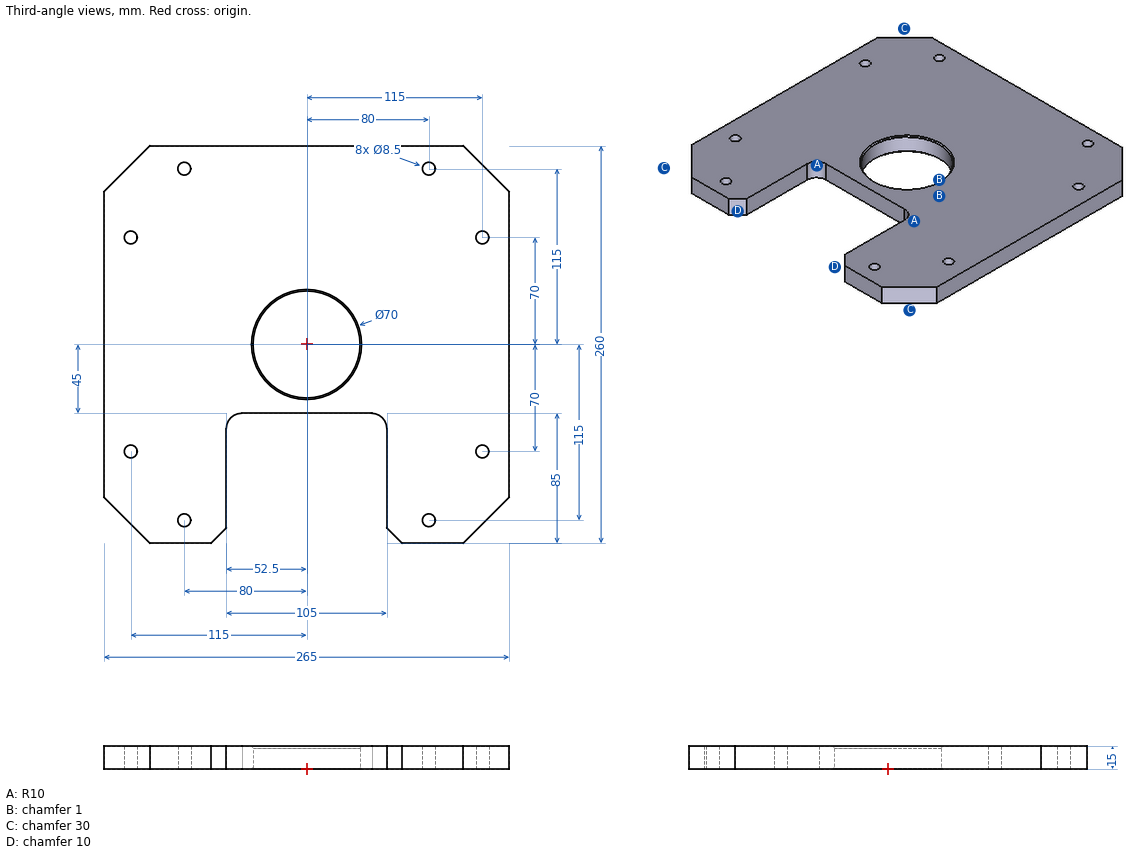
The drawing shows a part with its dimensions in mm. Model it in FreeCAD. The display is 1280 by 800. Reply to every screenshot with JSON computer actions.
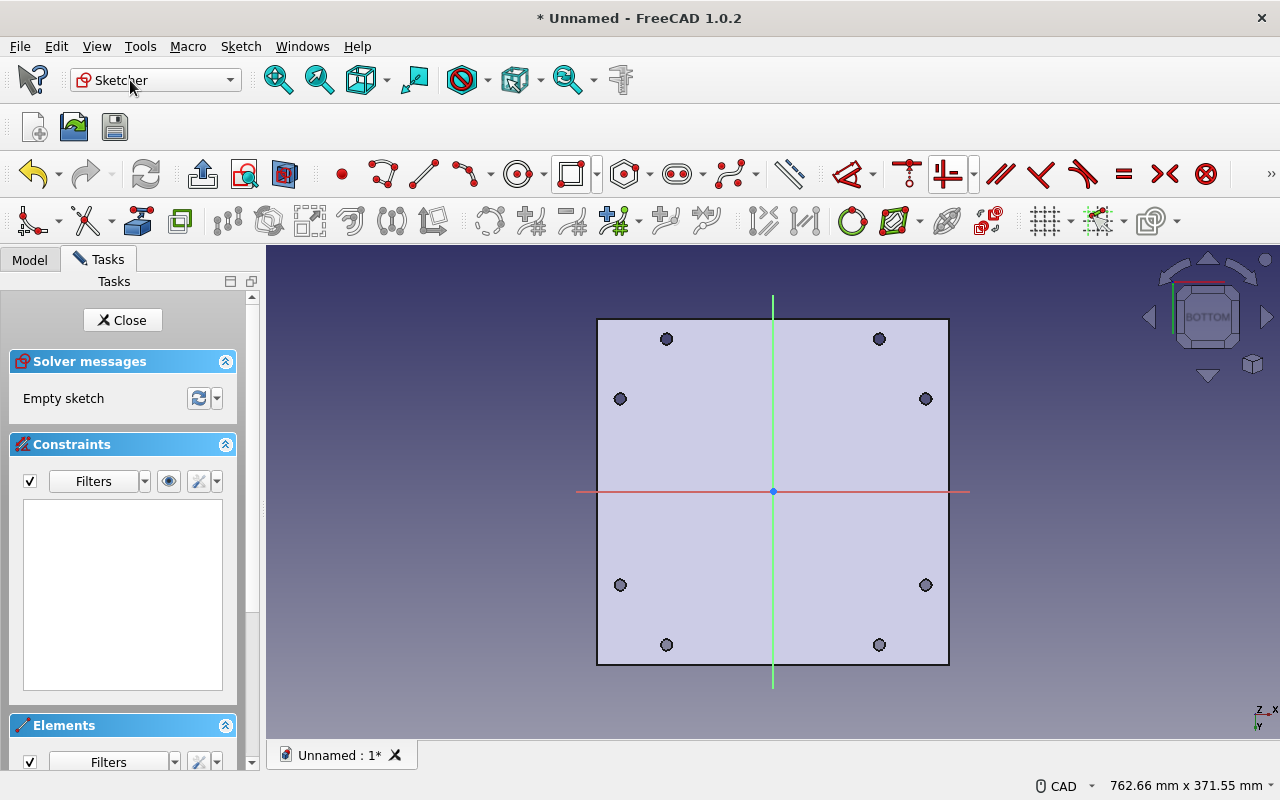
{"action": "scroll", "coordinate": [856, 300], "scroll_direction": "up", "scroll_amount": 3}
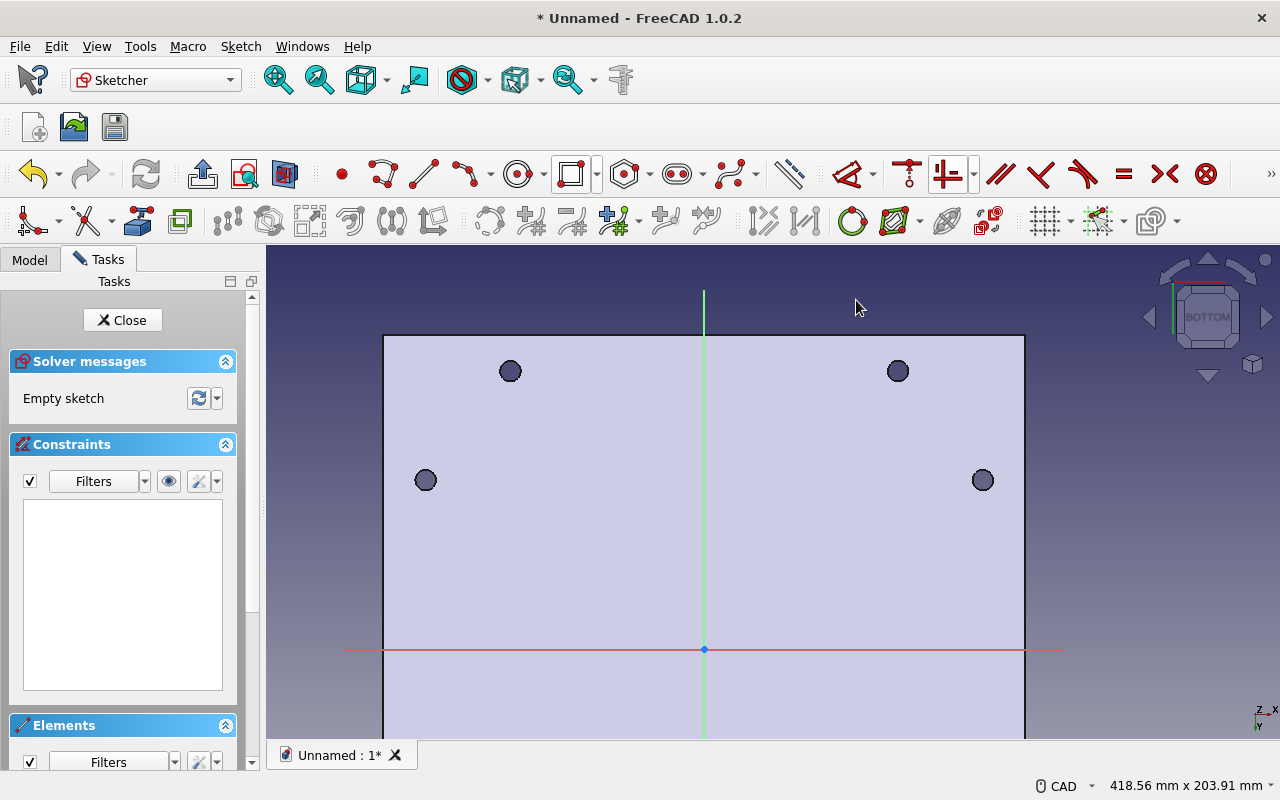
{"action": "key", "text": "g r"}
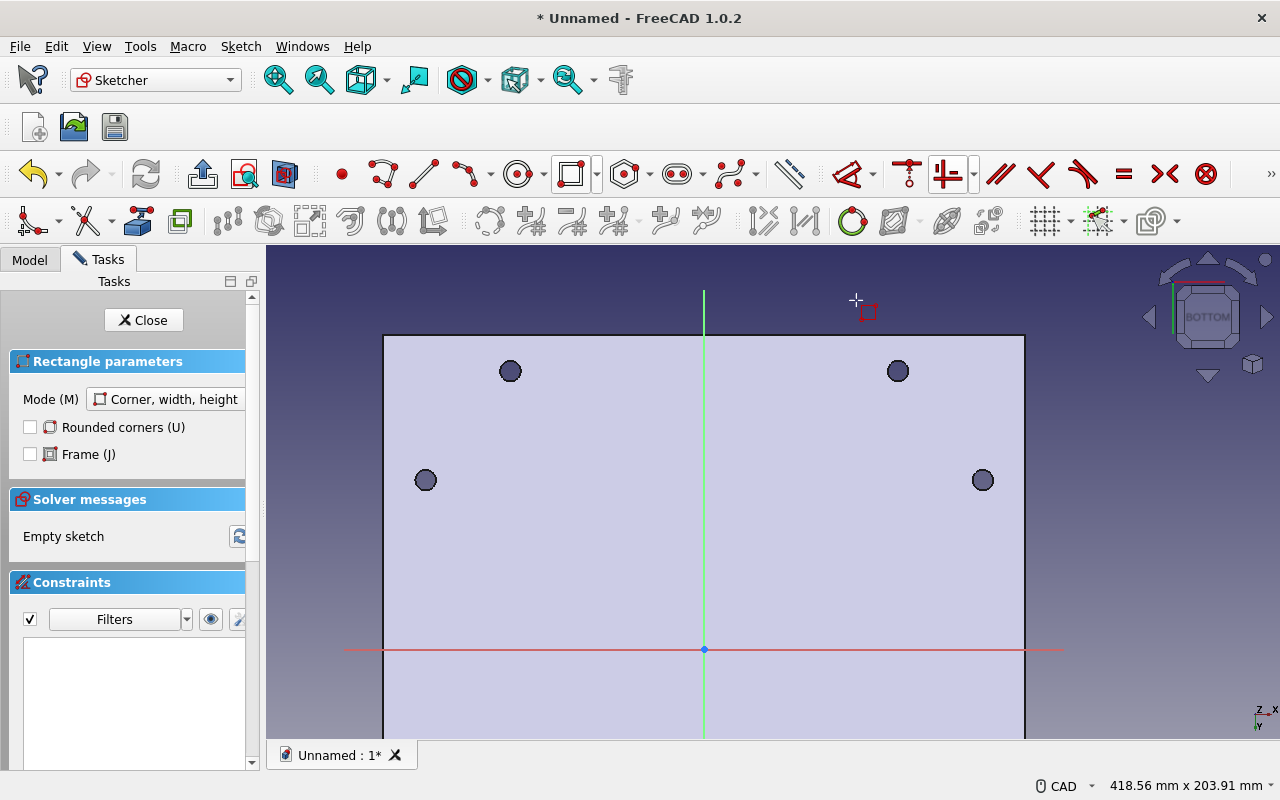
{"action": "left_click", "coordinate": [577, 335]}
{"action": "mouse_move", "coordinate": [831, 541]}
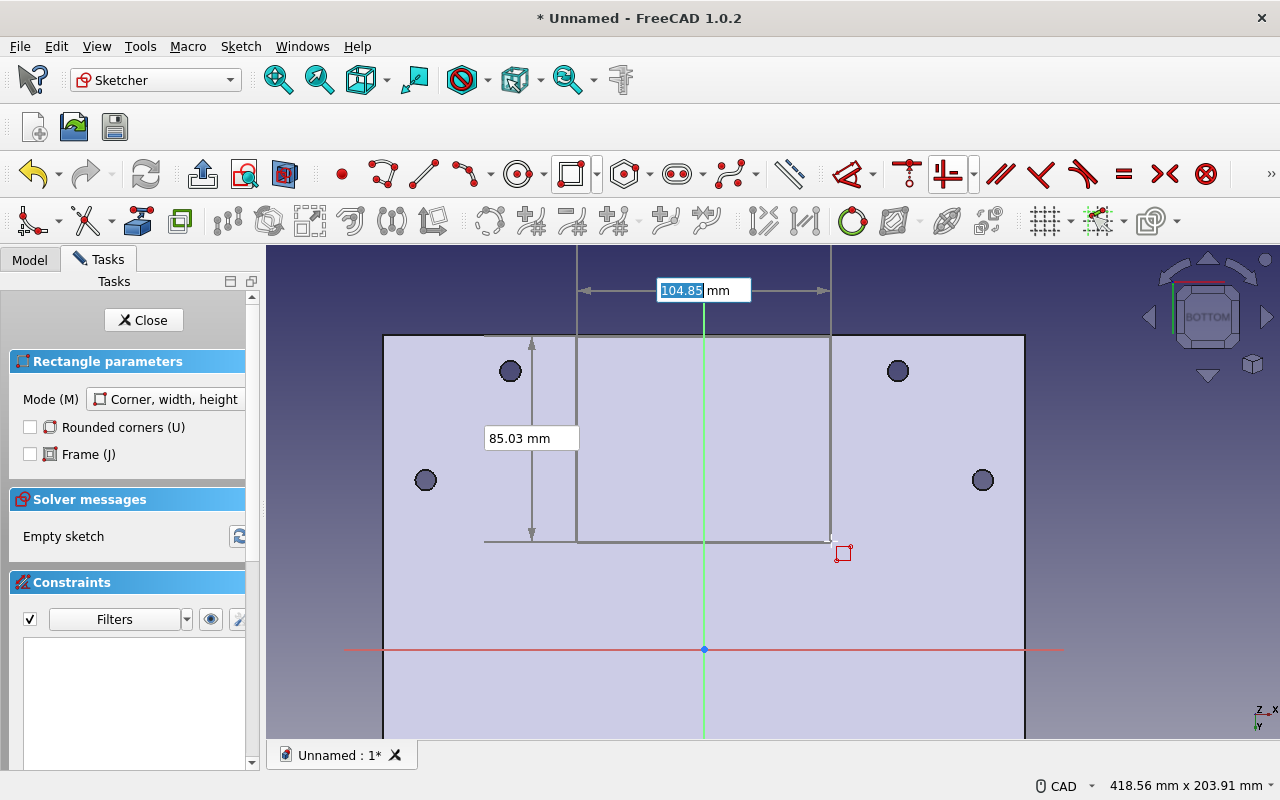
{"action": "type", "text": "105"}
{"action": "key", "text": "Tab"}
{"action": "type", "text": "85"}
{"action": "key", "text": "Return"}
{"action": "key", "text": "Escape"}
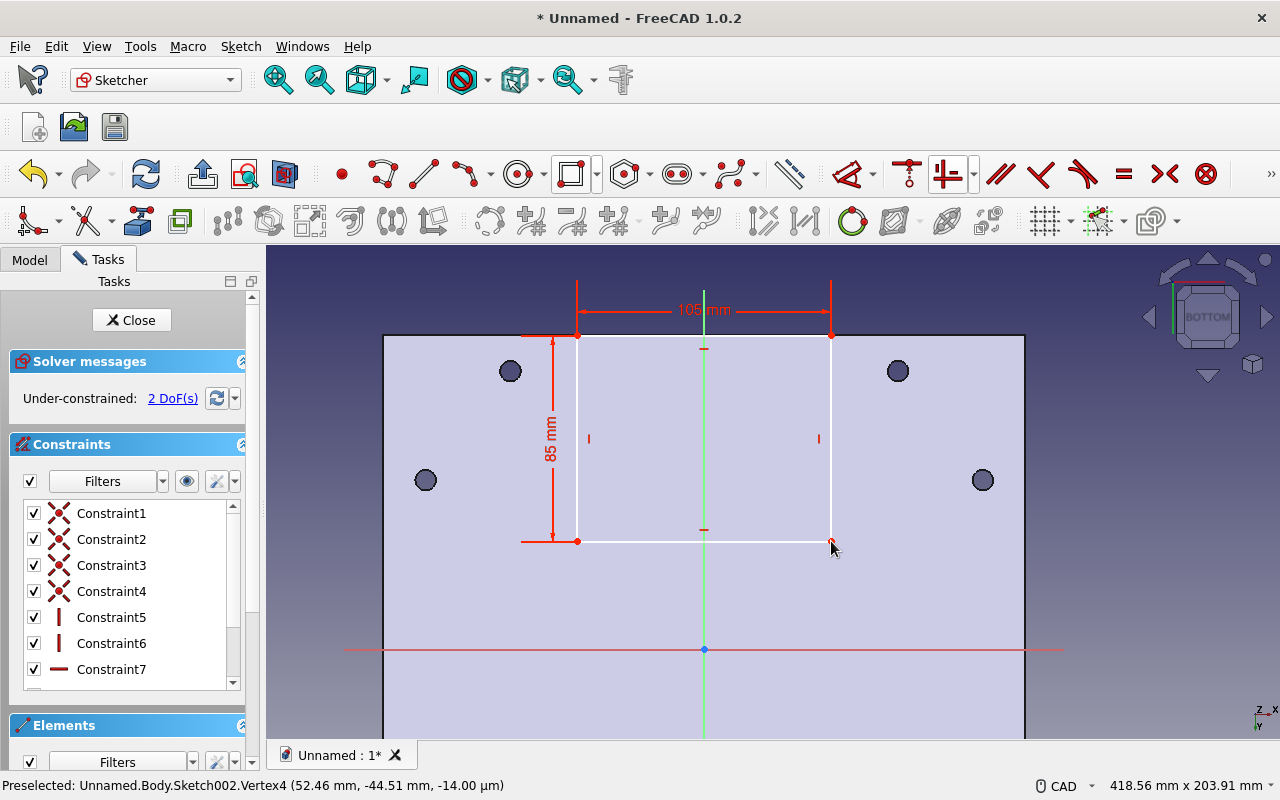
{"action": "key", "text": "d"}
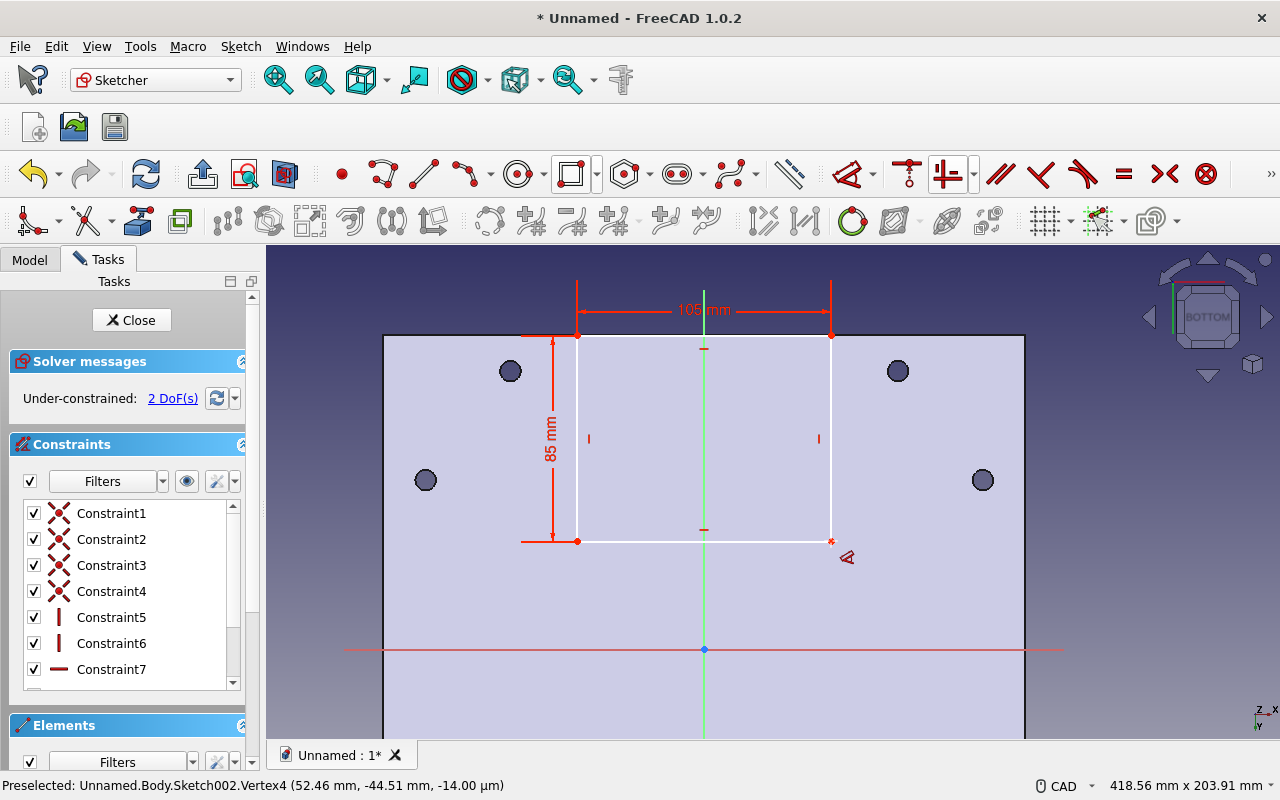
{"action": "left_click", "coordinate": [577, 542]}
{"action": "left_click", "coordinate": [543, 596]}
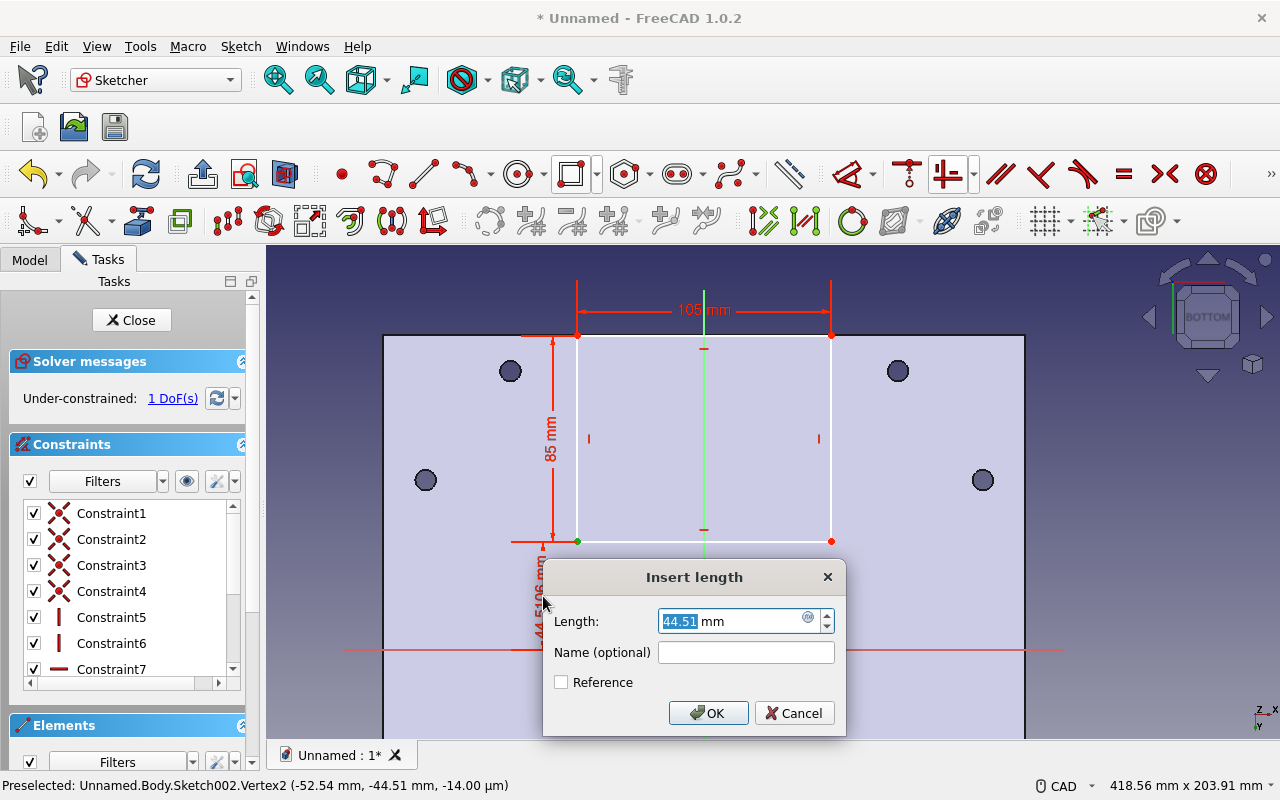
{"action": "type", "text": "45"}
{"action": "key", "text": "Return"}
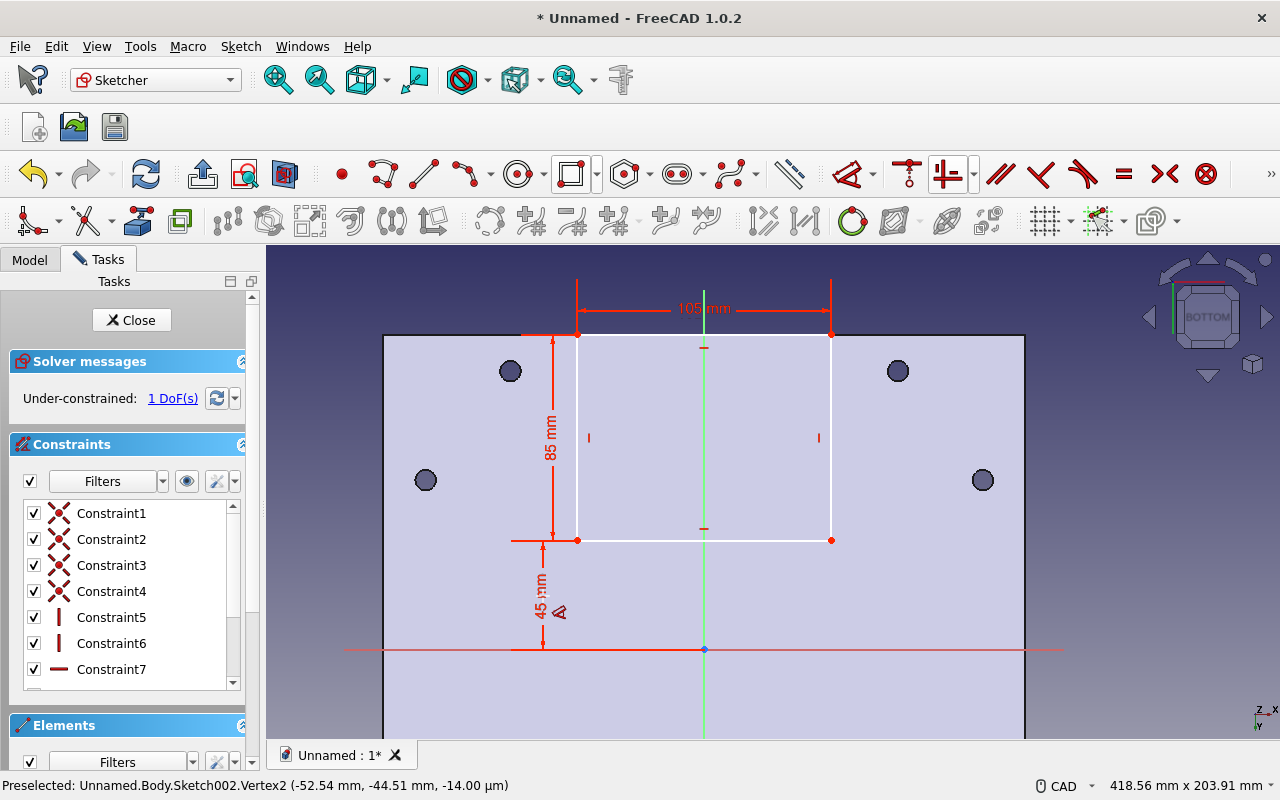
{"action": "left_click", "coordinate": [577, 335]}
{"action": "left_click", "coordinate": [641, 684]}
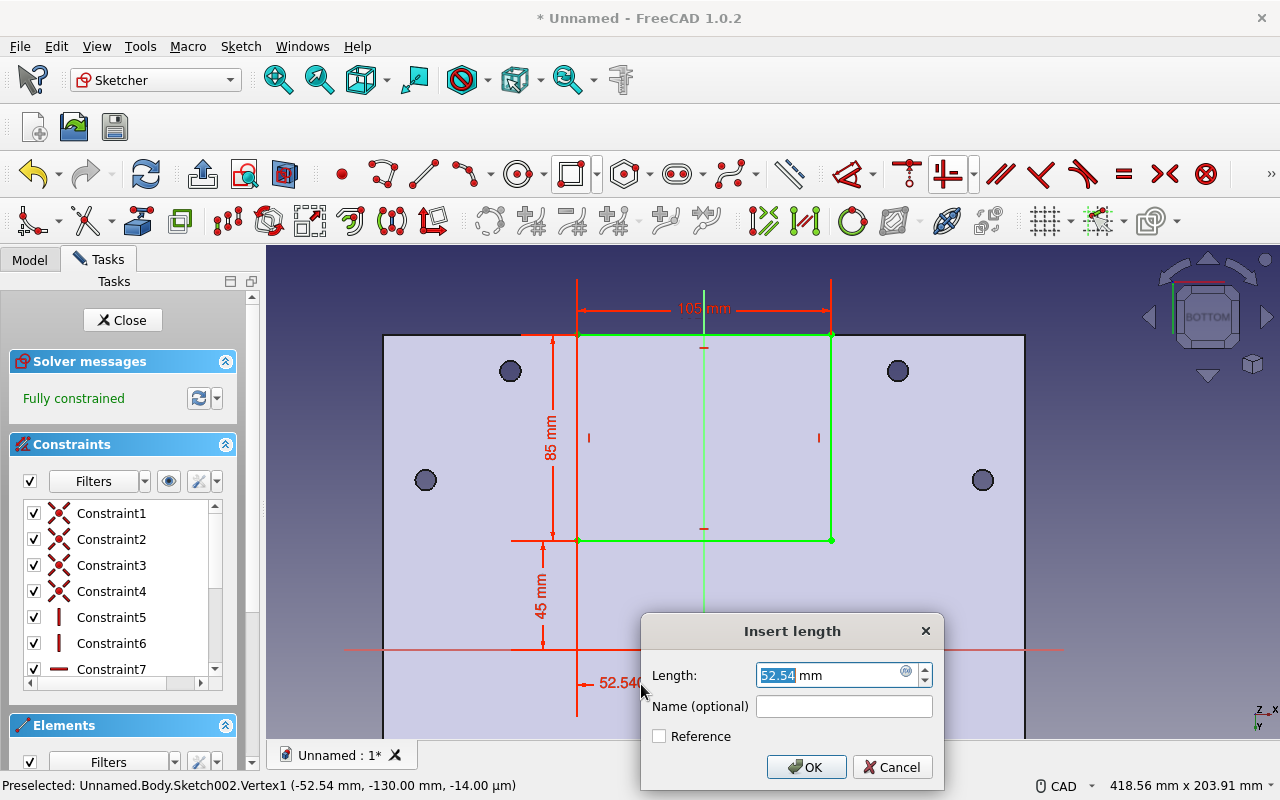
{"action": "type", "text": "52.5"}
{"action": "key", "text": "Return"}
{"action": "key", "text": "Escape"}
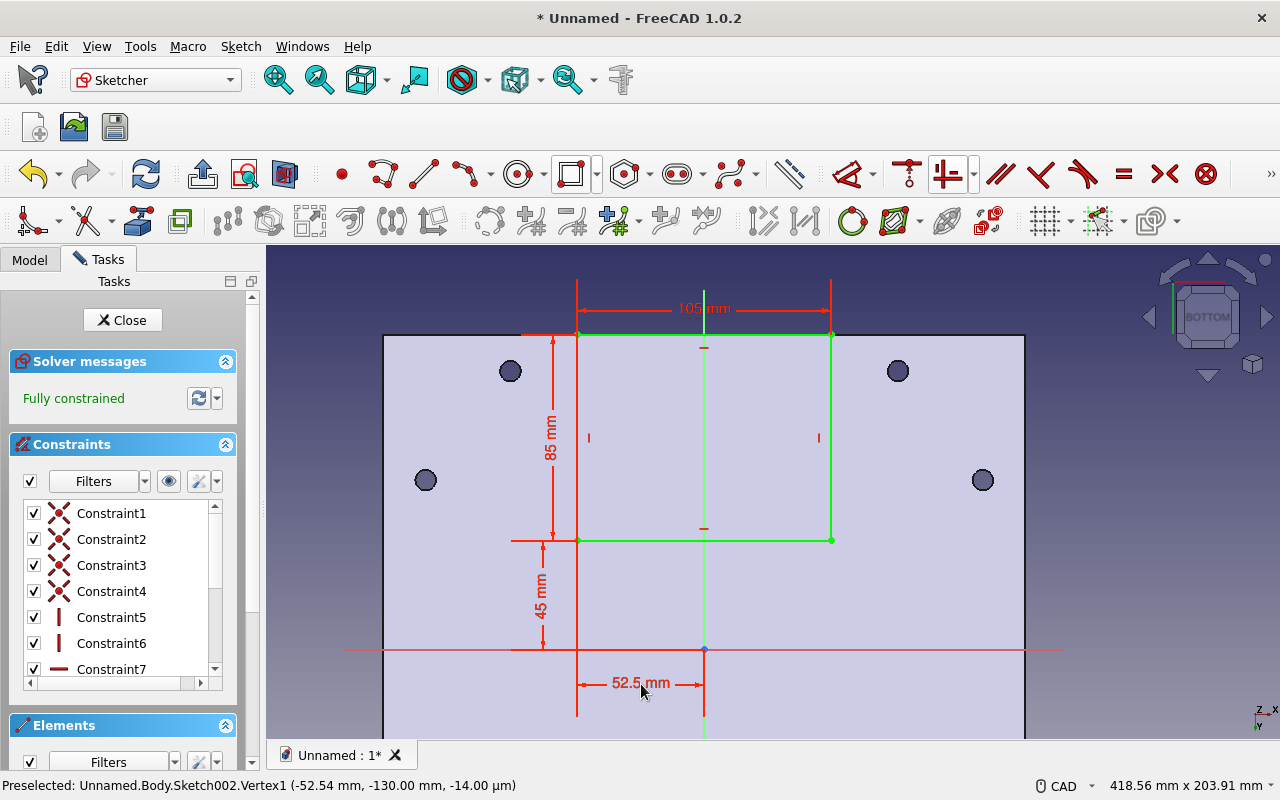
{"action": "left_click", "coordinate": [123, 320]}